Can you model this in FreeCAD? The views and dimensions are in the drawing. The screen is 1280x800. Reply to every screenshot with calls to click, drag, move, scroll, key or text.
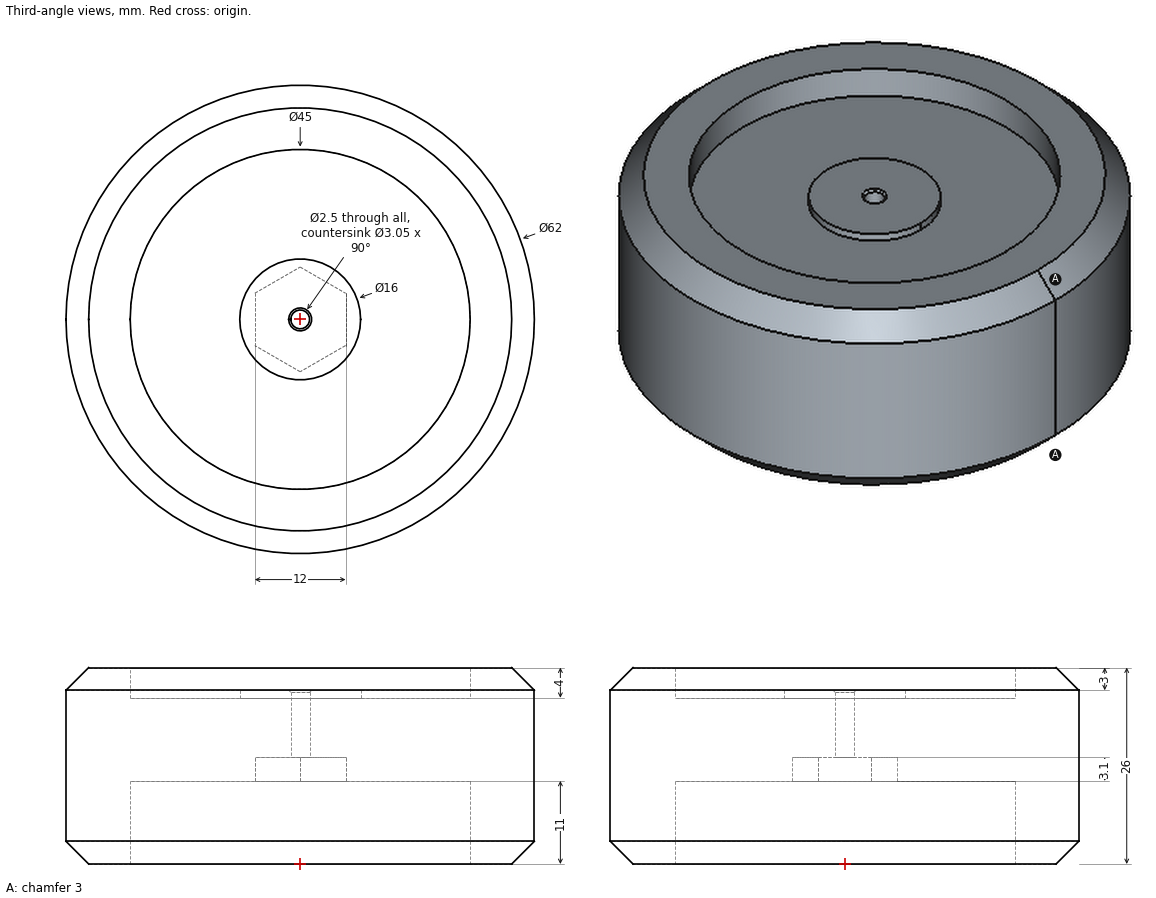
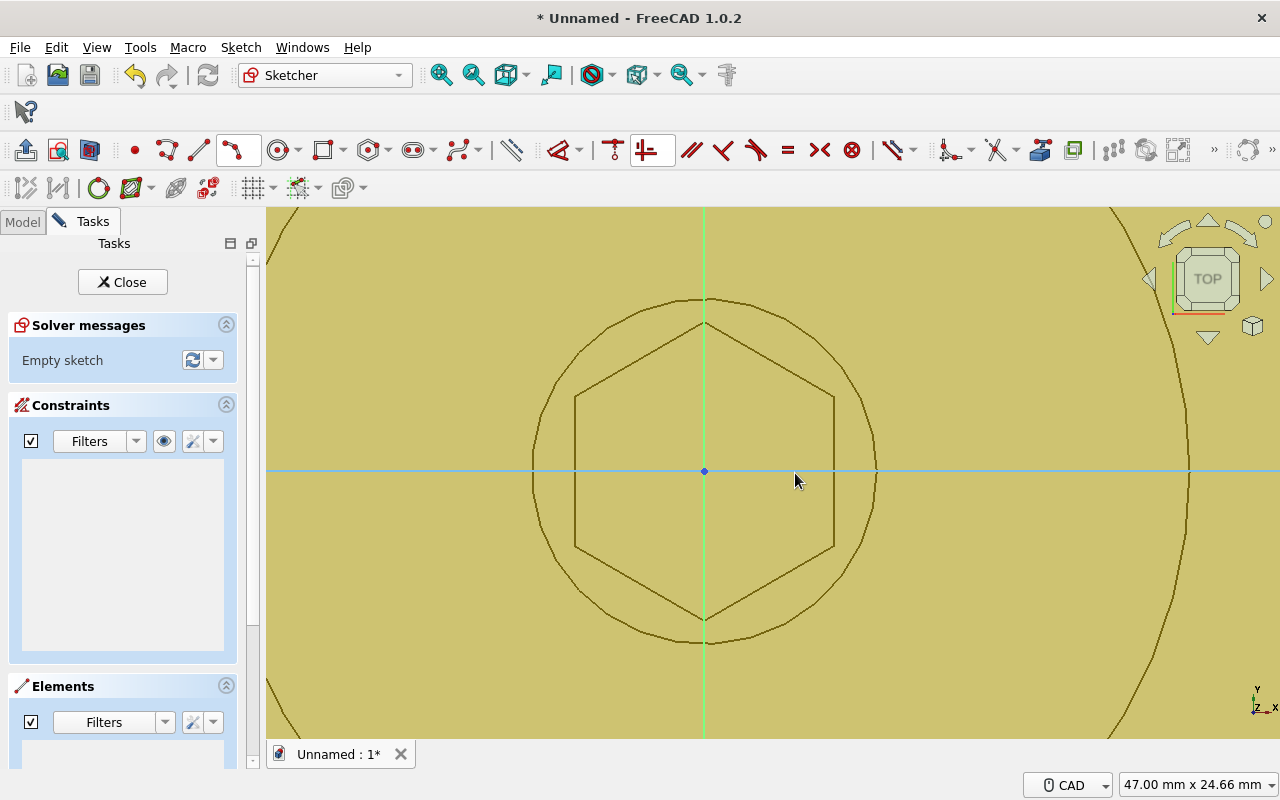
click(278, 150)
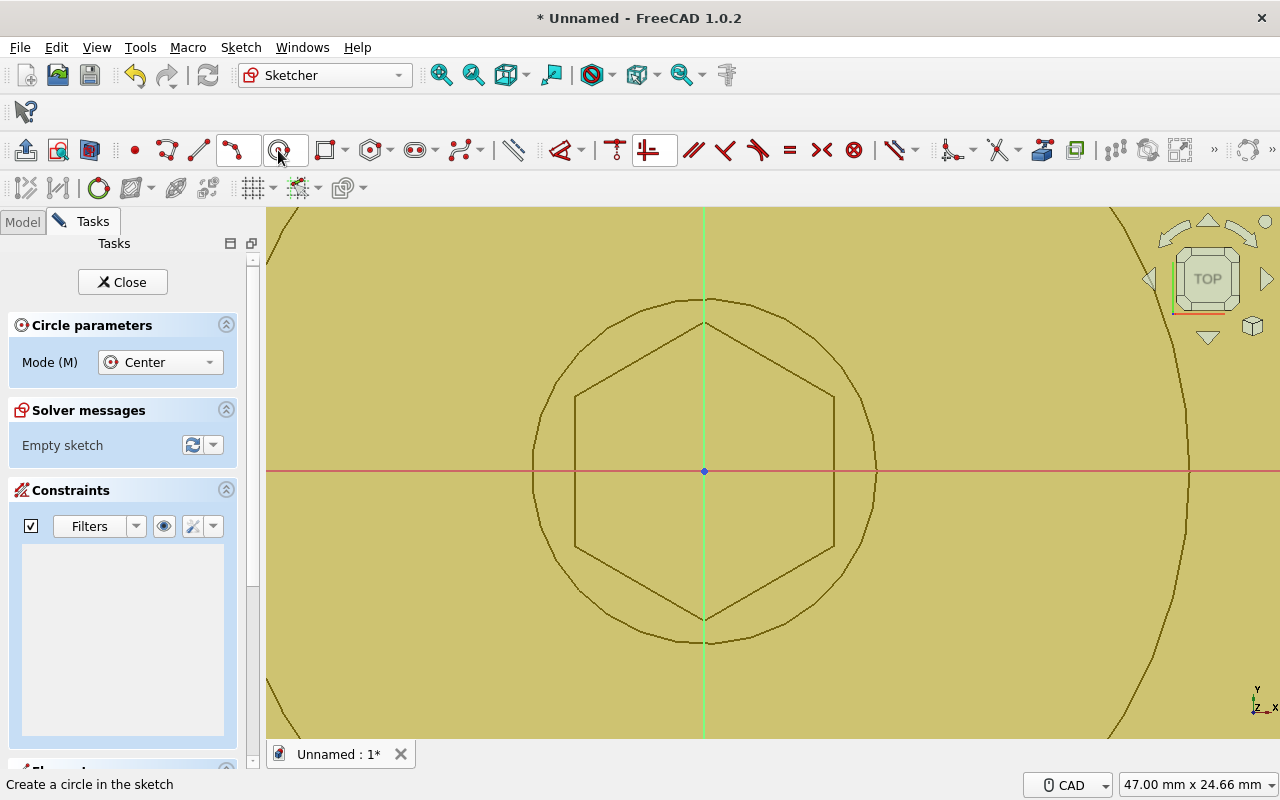
click(704, 471)
click(826, 349)
key(Escape)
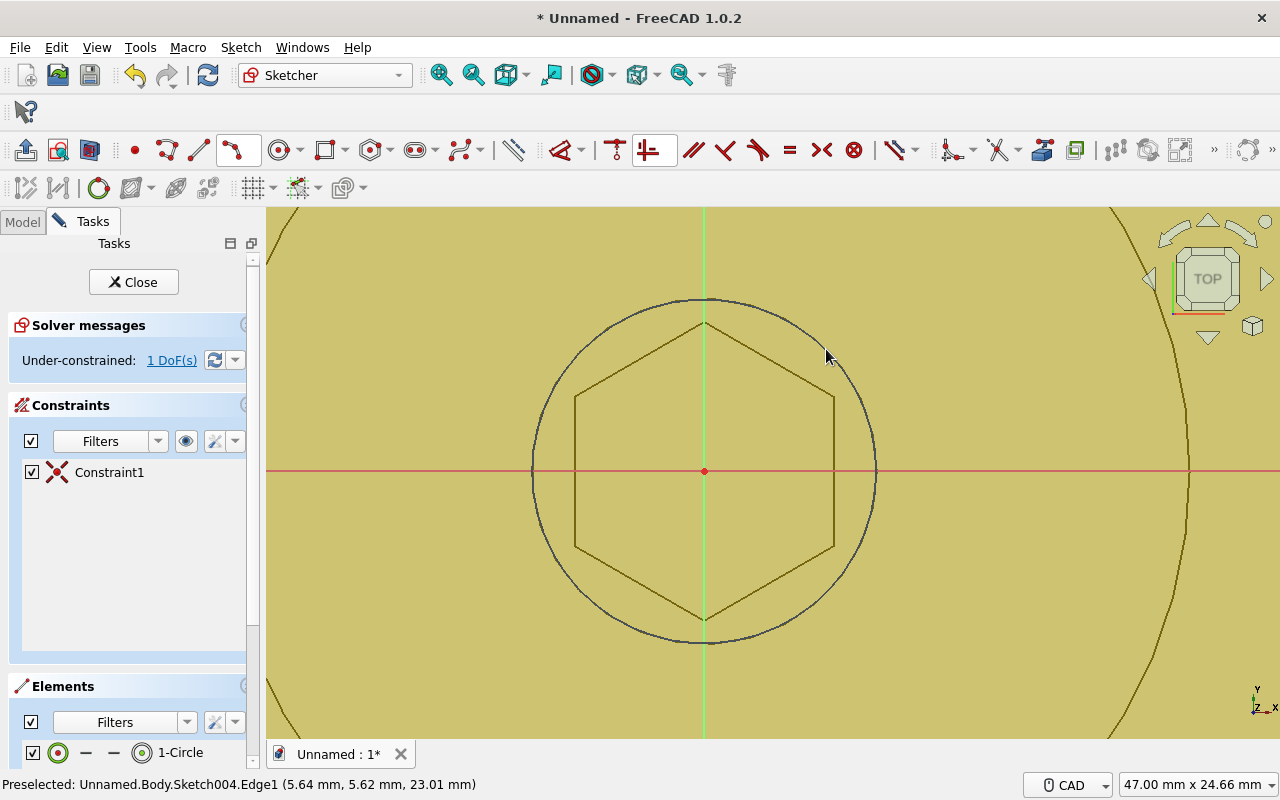
click(560, 150)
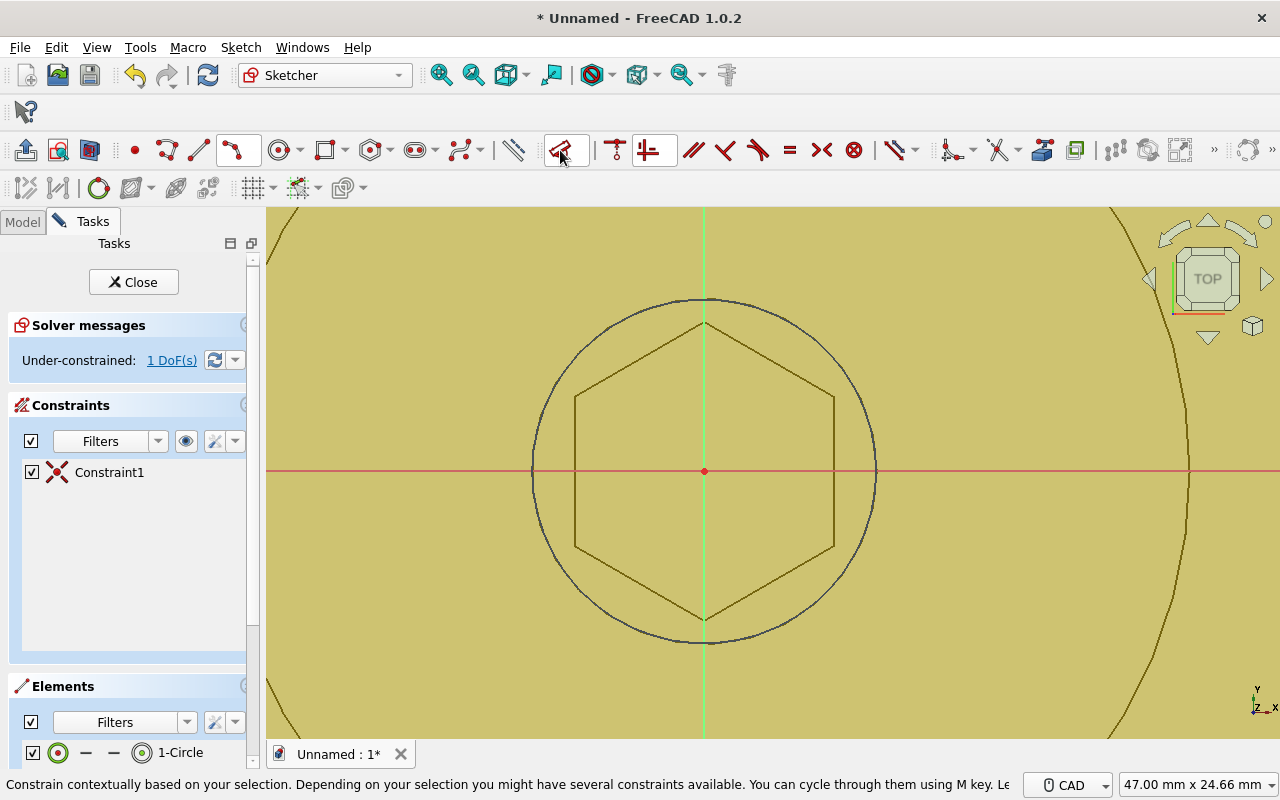
click(825, 349)
click(847, 326)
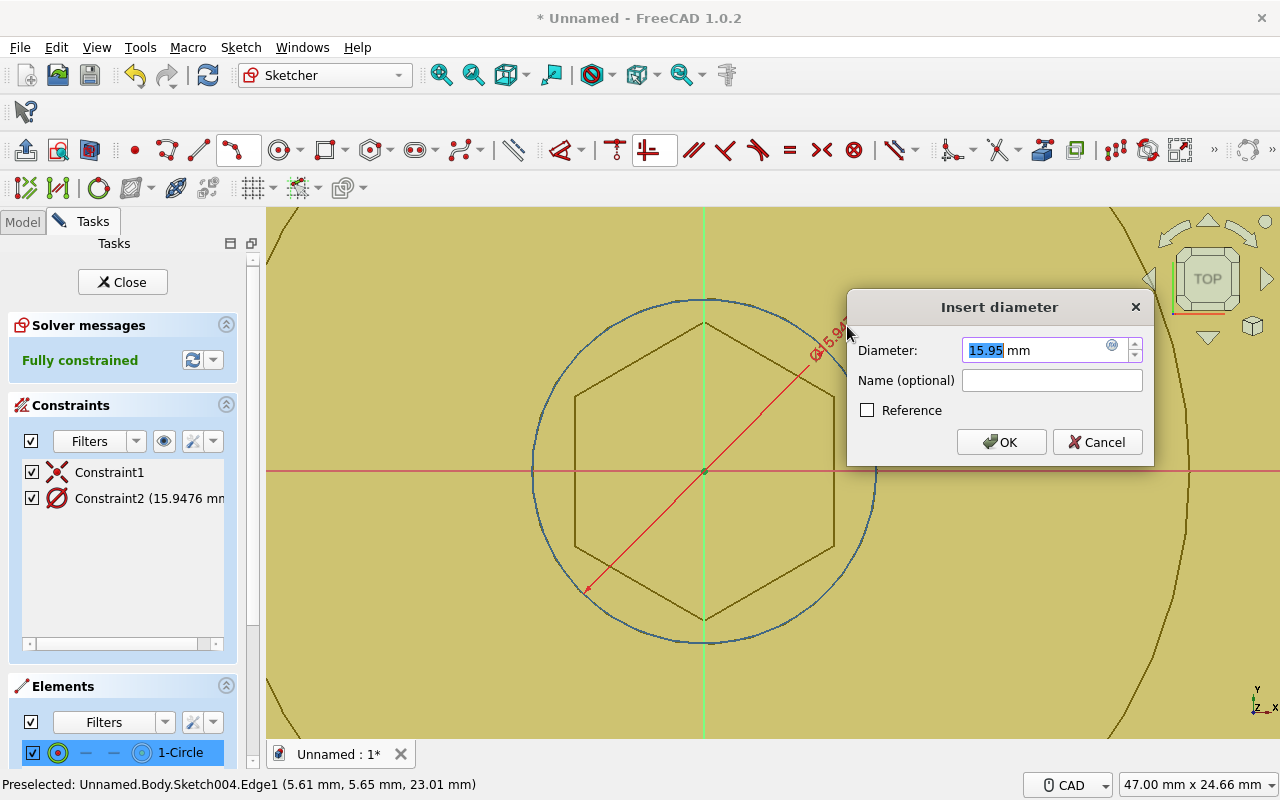
text(16)
key(Return)
key(Escape)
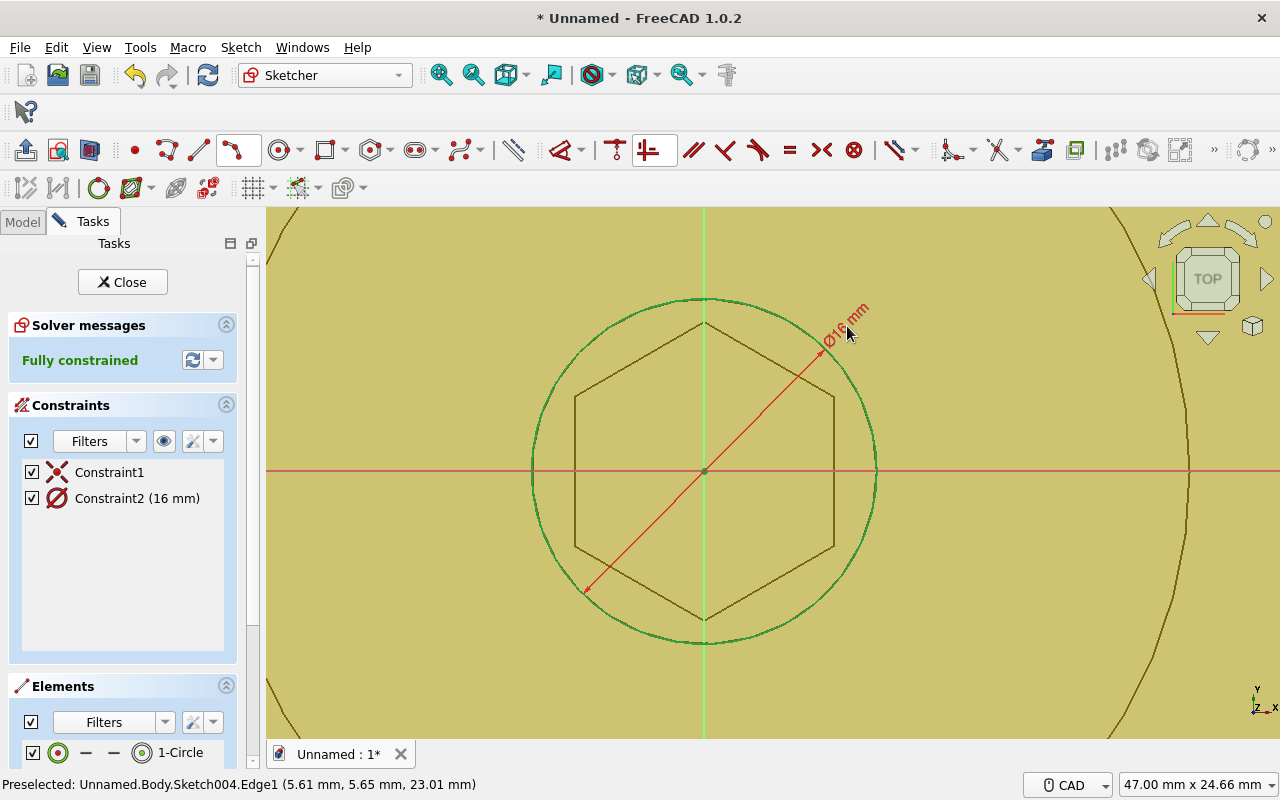
click(123, 282)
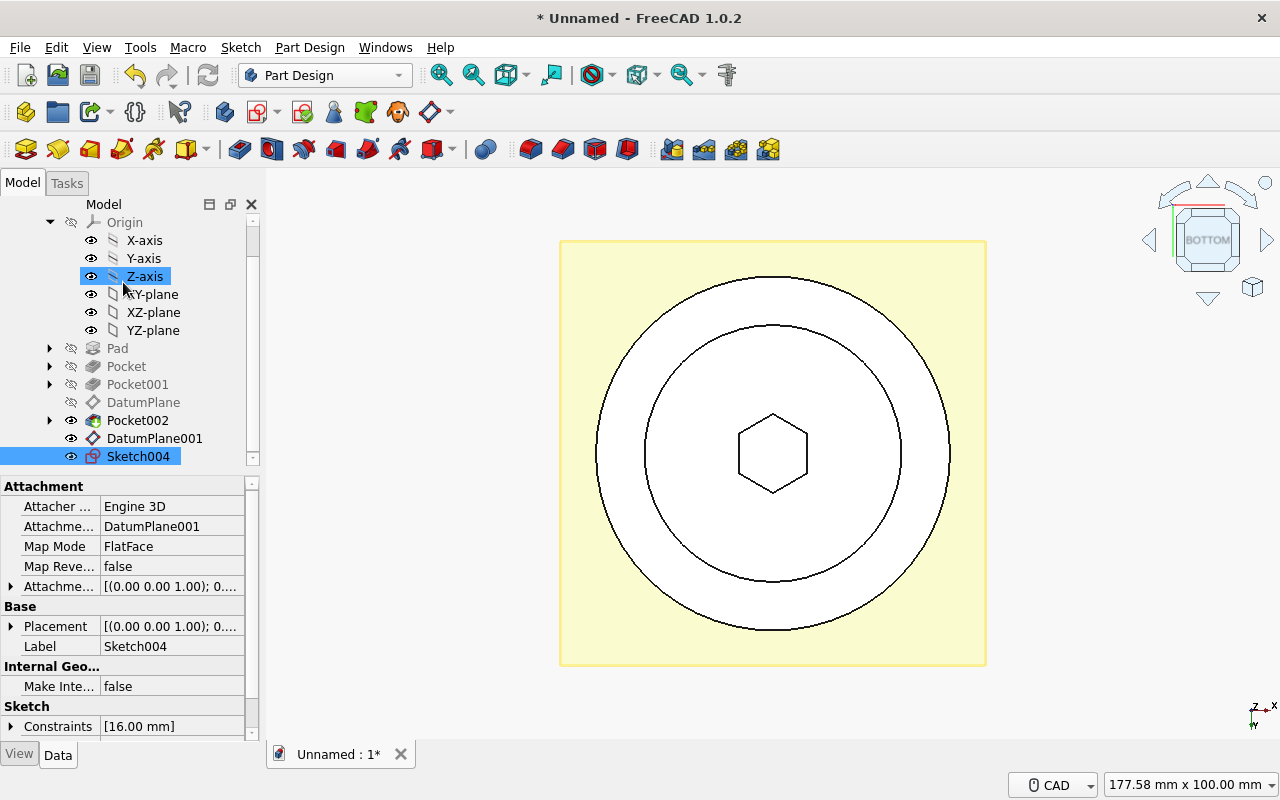
click(240, 150)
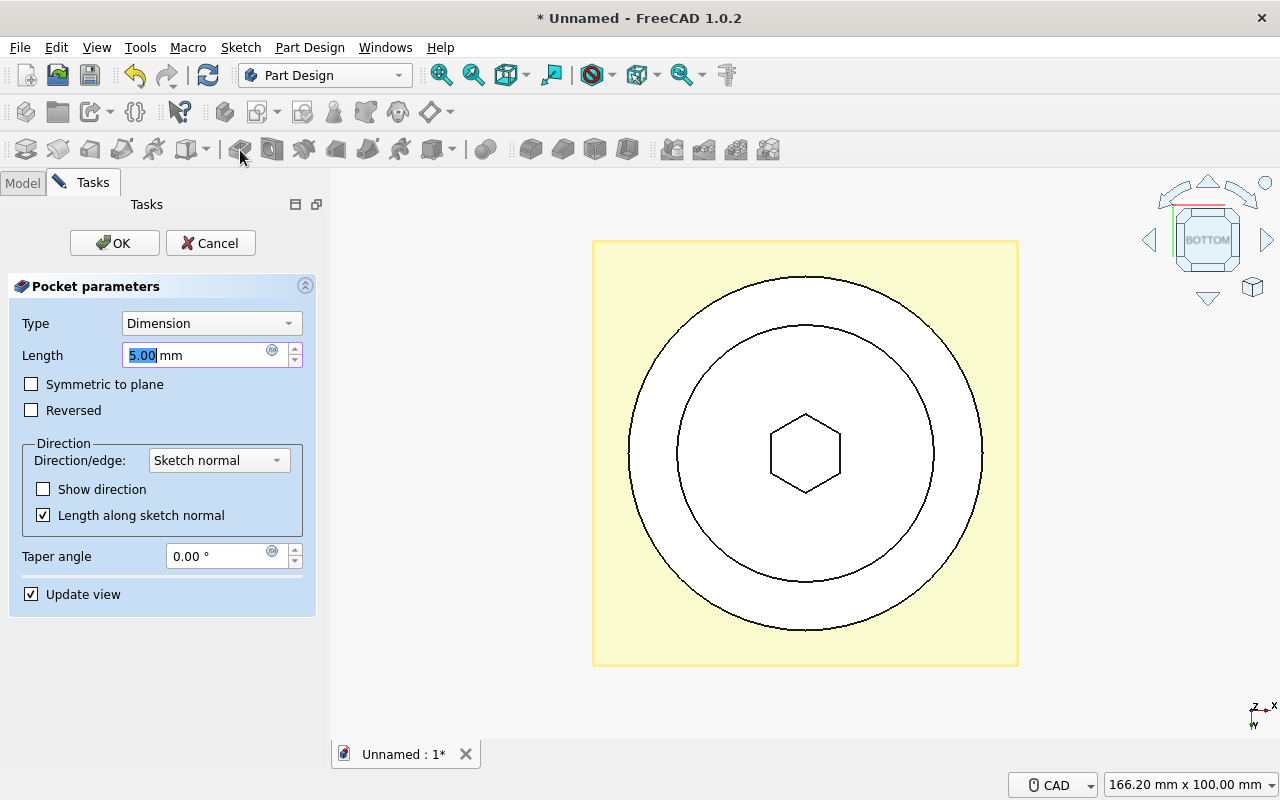
text(3)
key(Tab)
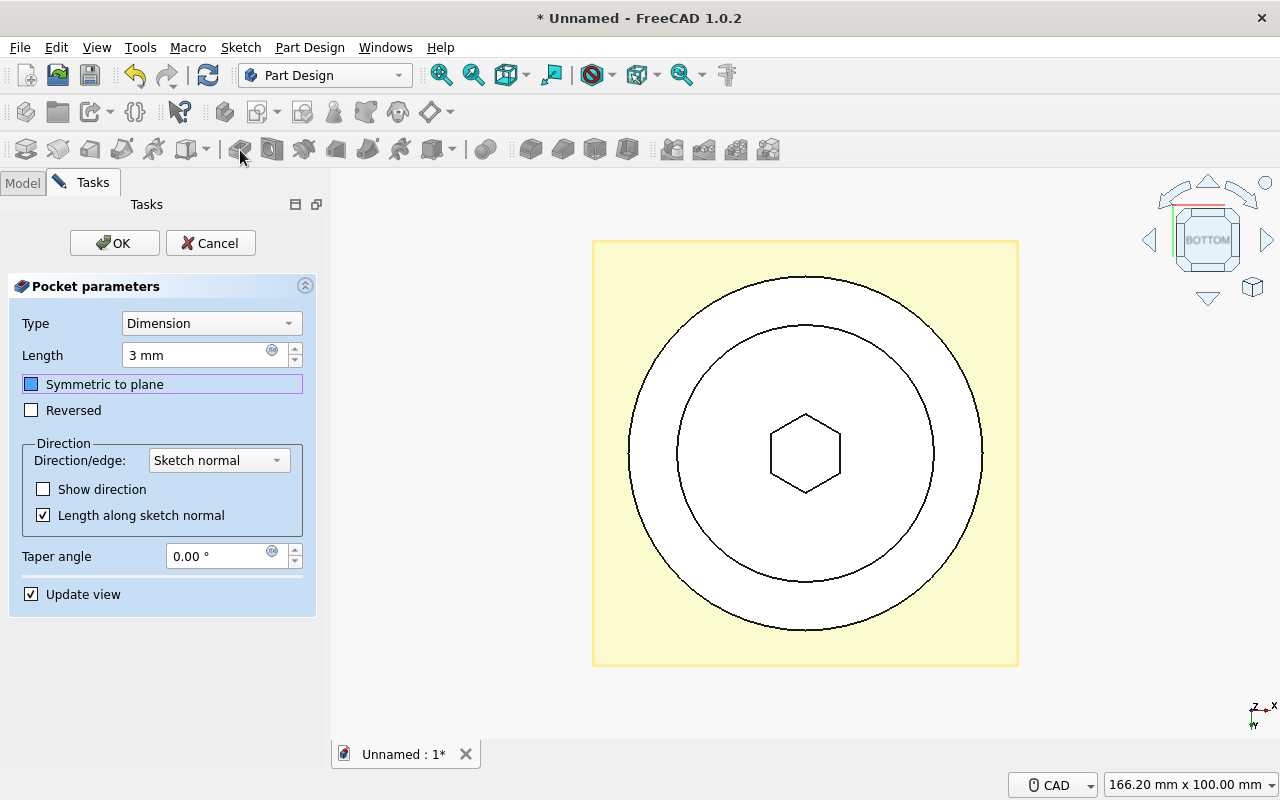
click(30, 410)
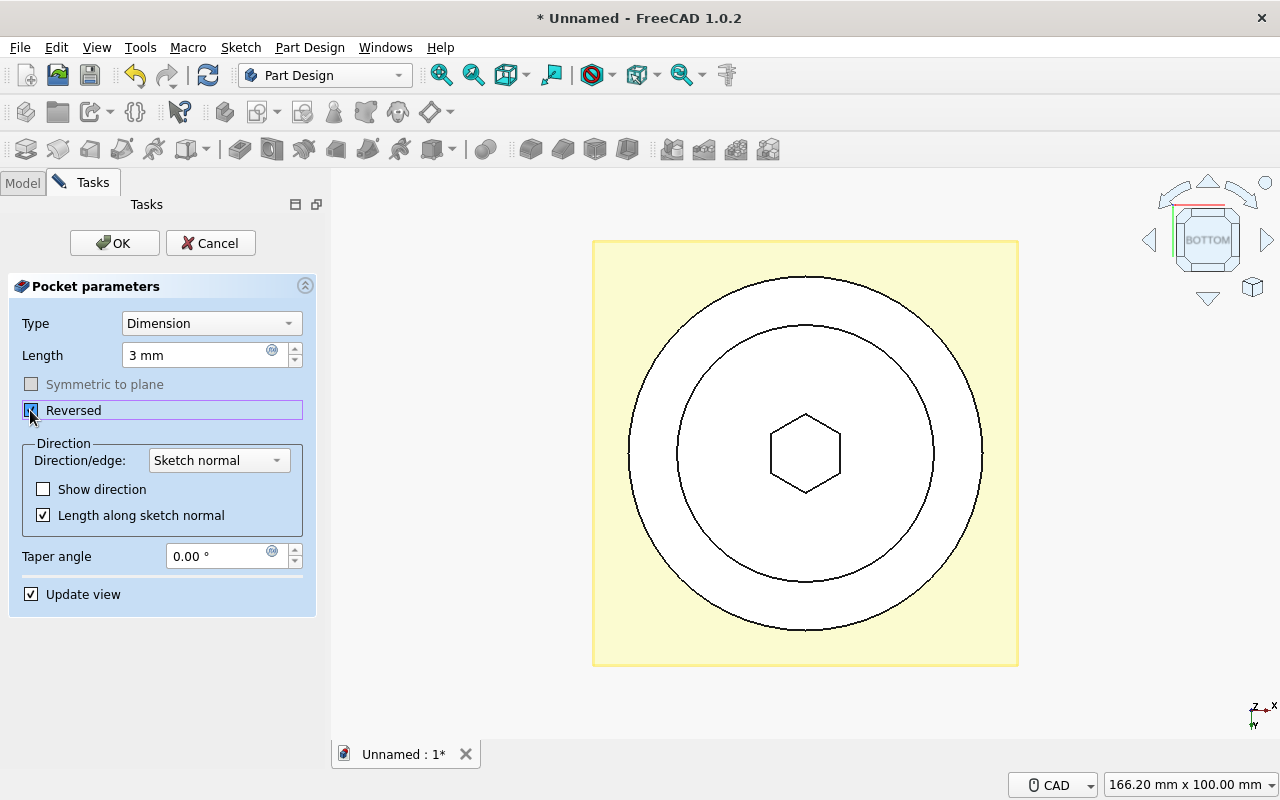
click(115, 243)